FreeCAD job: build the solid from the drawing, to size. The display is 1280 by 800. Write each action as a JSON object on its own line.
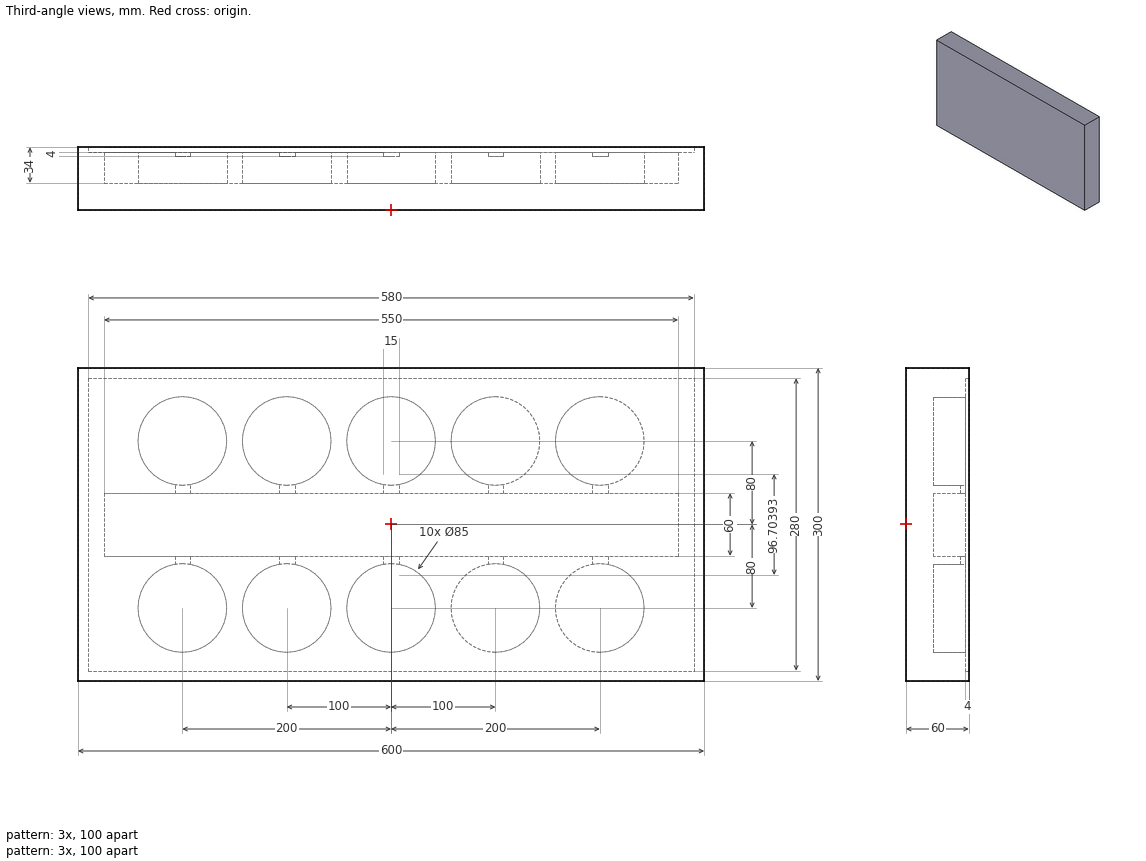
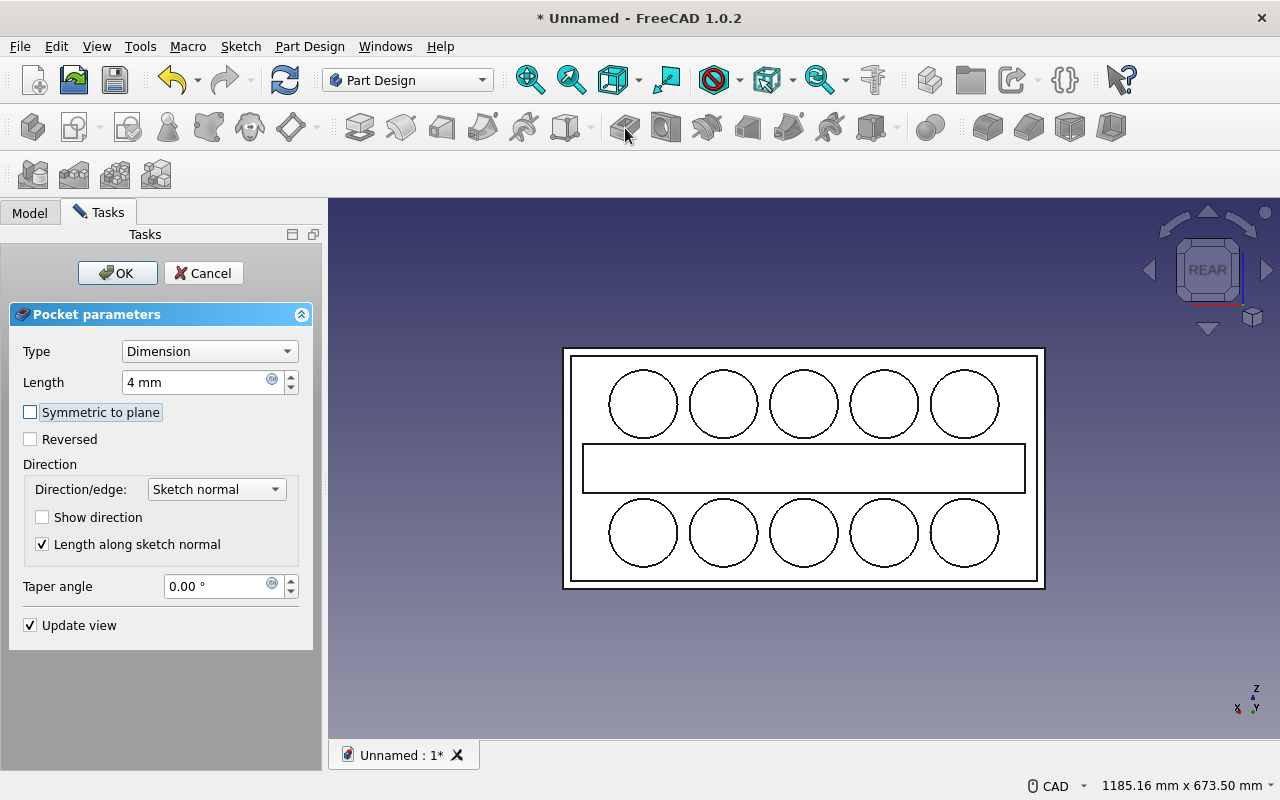
{"action": "left_click", "coordinate": [118, 273]}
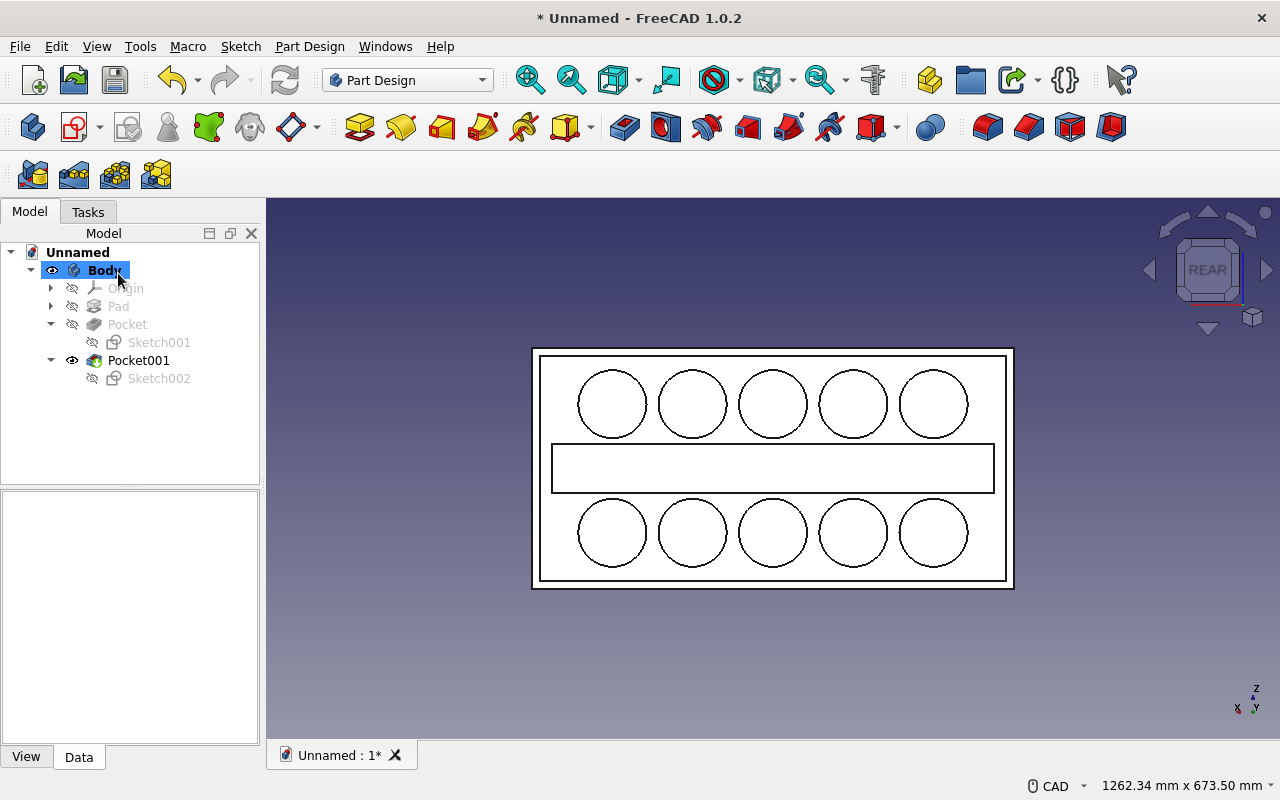
{"action": "left_click", "coordinate": [573, 371]}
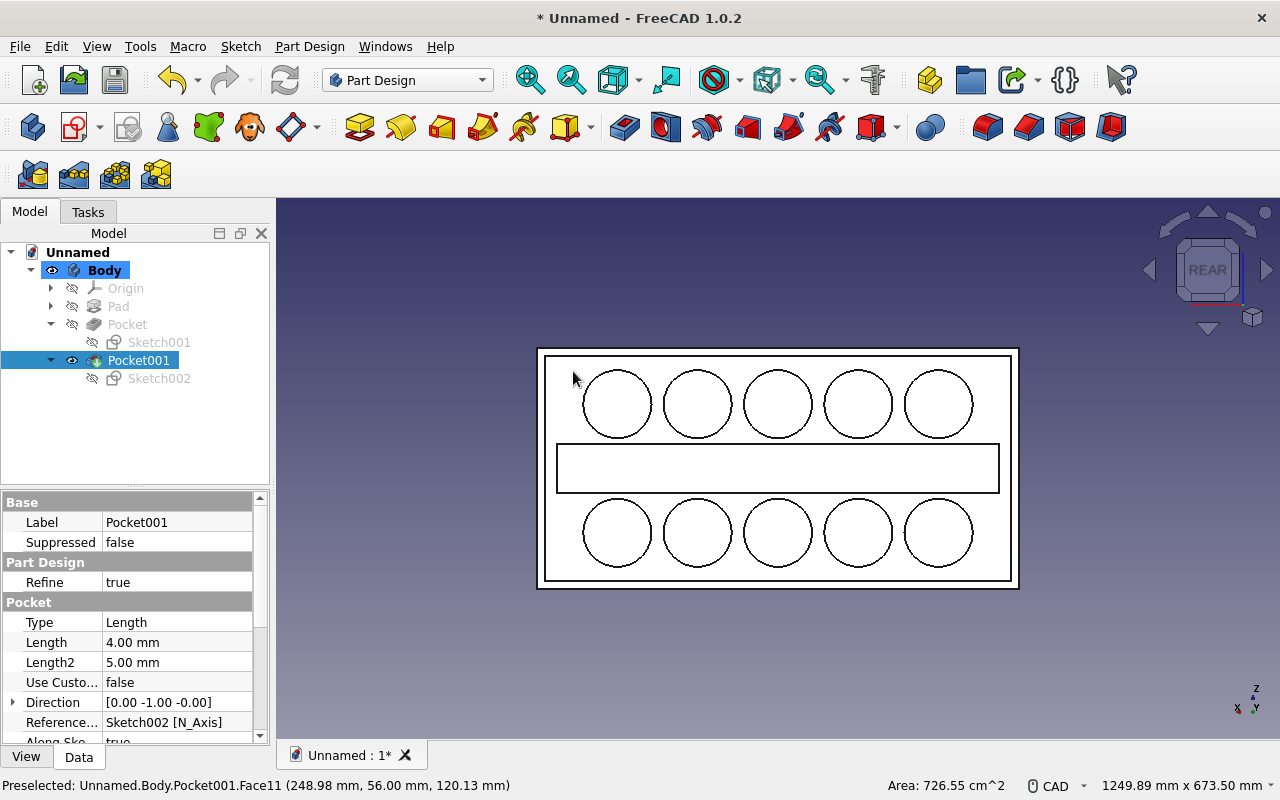
{"action": "left_click", "coordinate": [74, 128]}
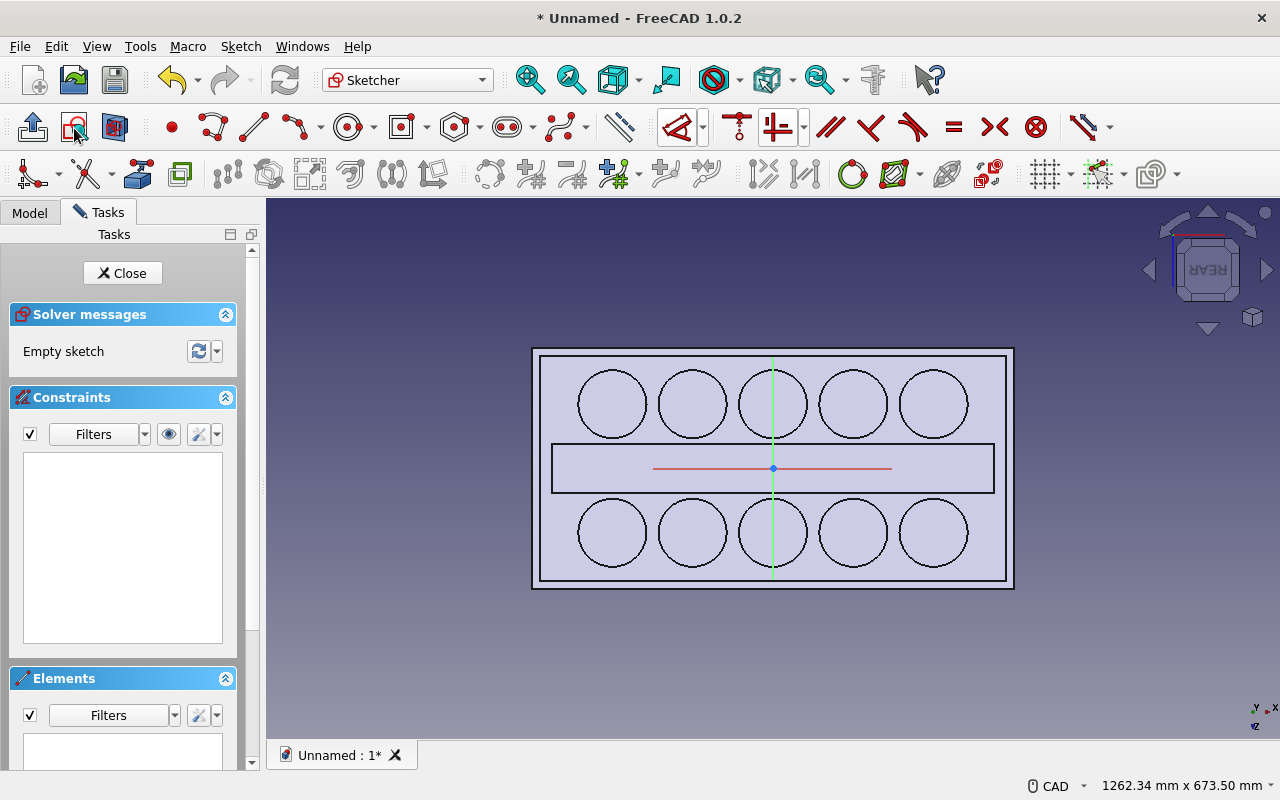
{"action": "left_click", "coordinate": [115, 128]}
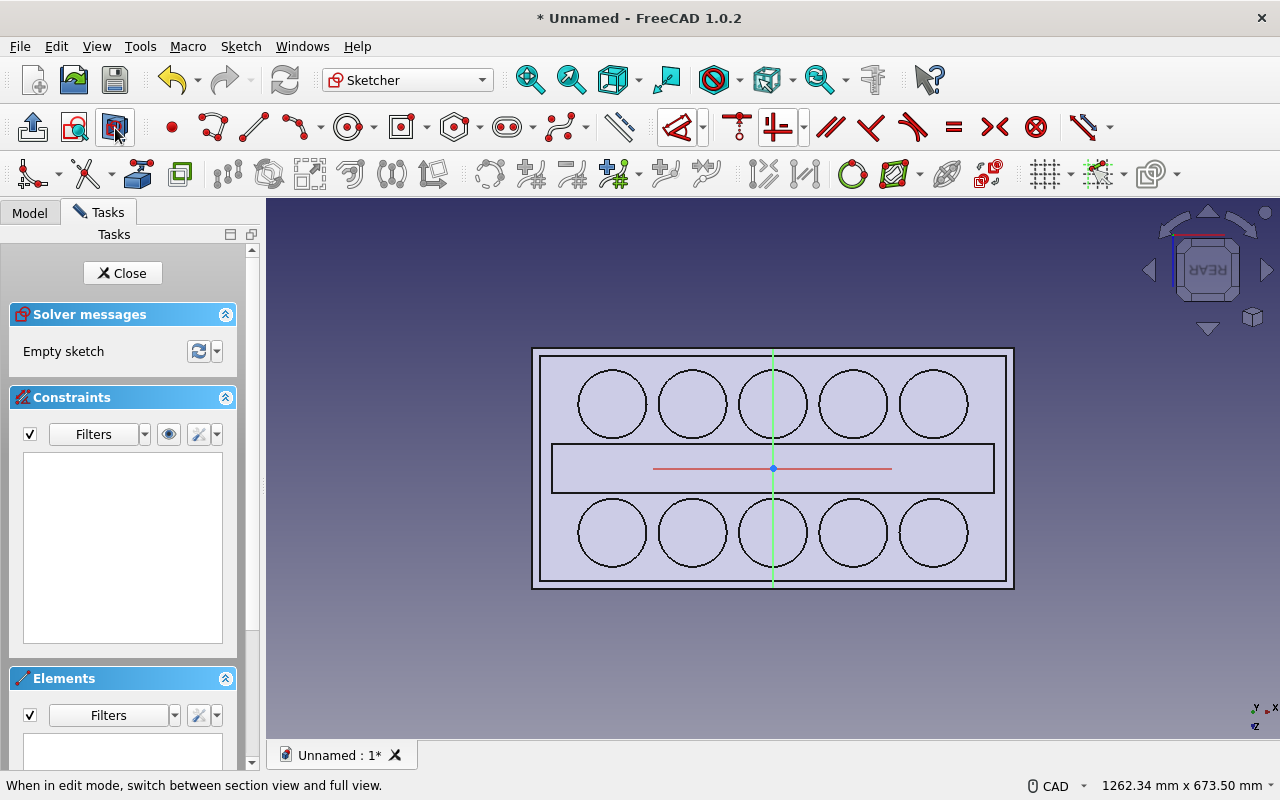
{"action": "scroll", "coordinate": [795, 468], "scroll_direction": "up", "scroll_amount": 7}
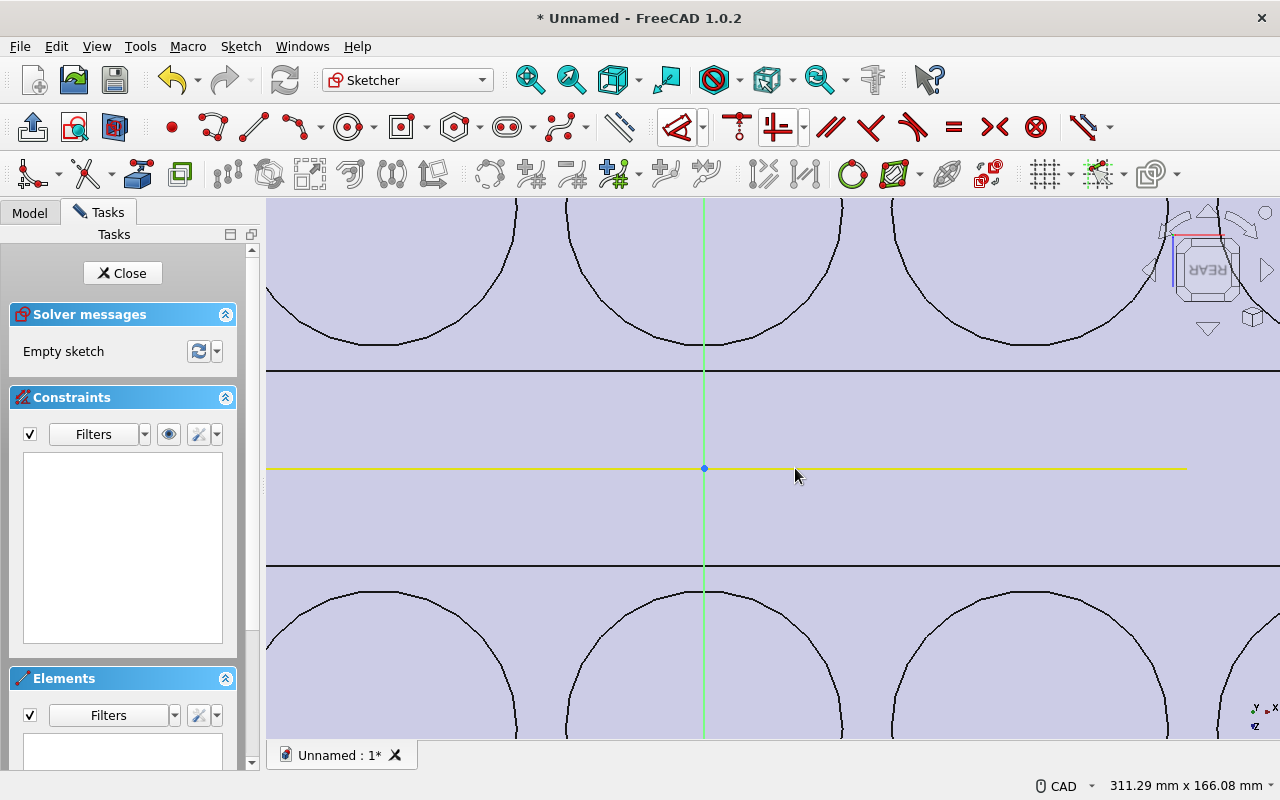
{"action": "left_click", "coordinate": [400, 128]}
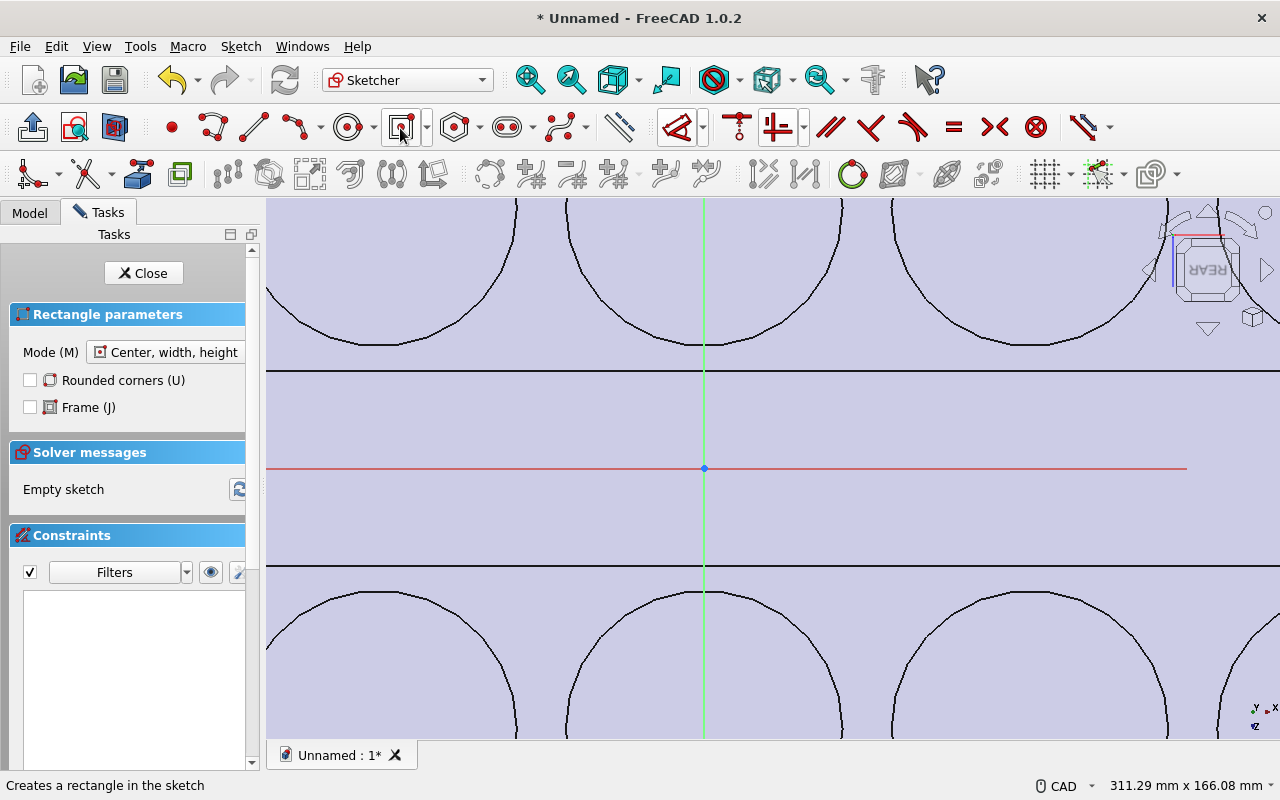
{"action": "left_click", "coordinate": [704, 468]}
{"action": "mouse_move", "coordinate": [729, 311]}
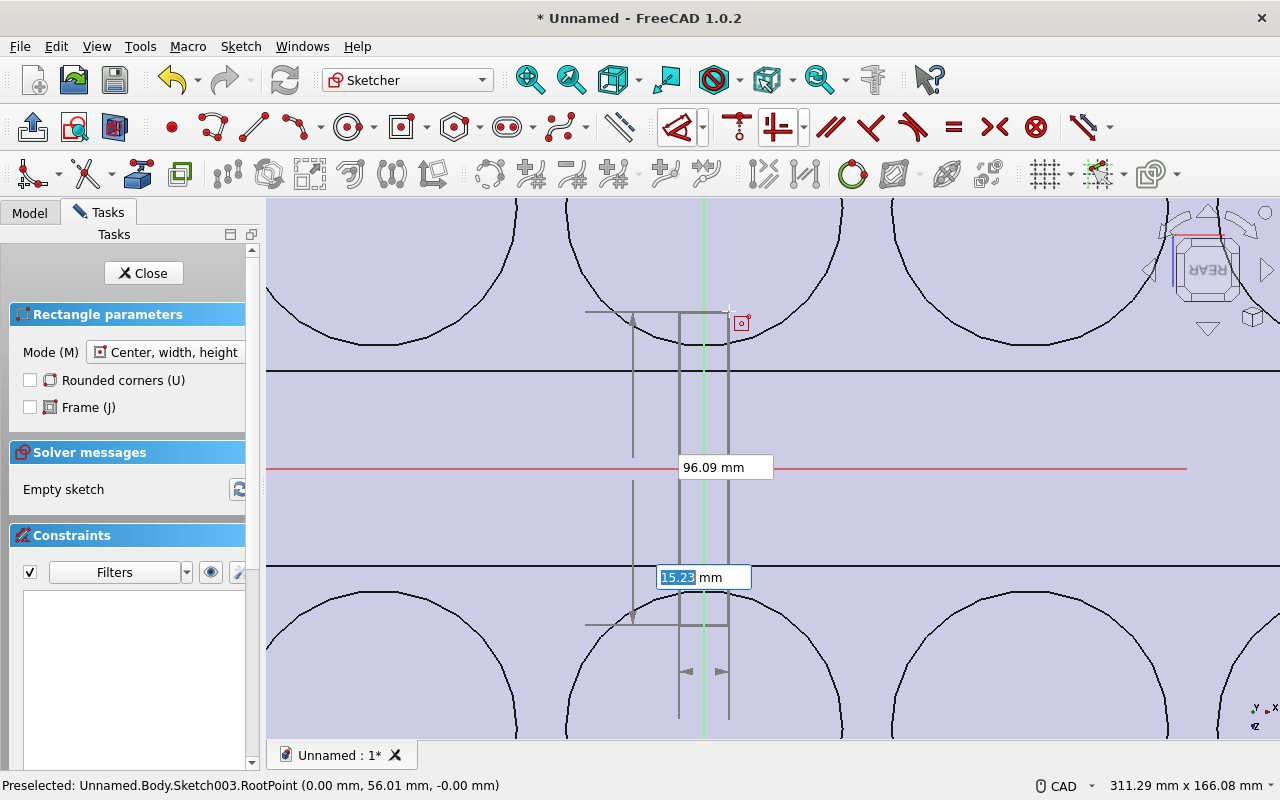
{"action": "type", "text": "15"}
{"action": "key", "text": "Tab"}
{"action": "type", "text": "96.70393"}
{"action": "key", "text": "Return"}
{"action": "key", "text": "Escape"}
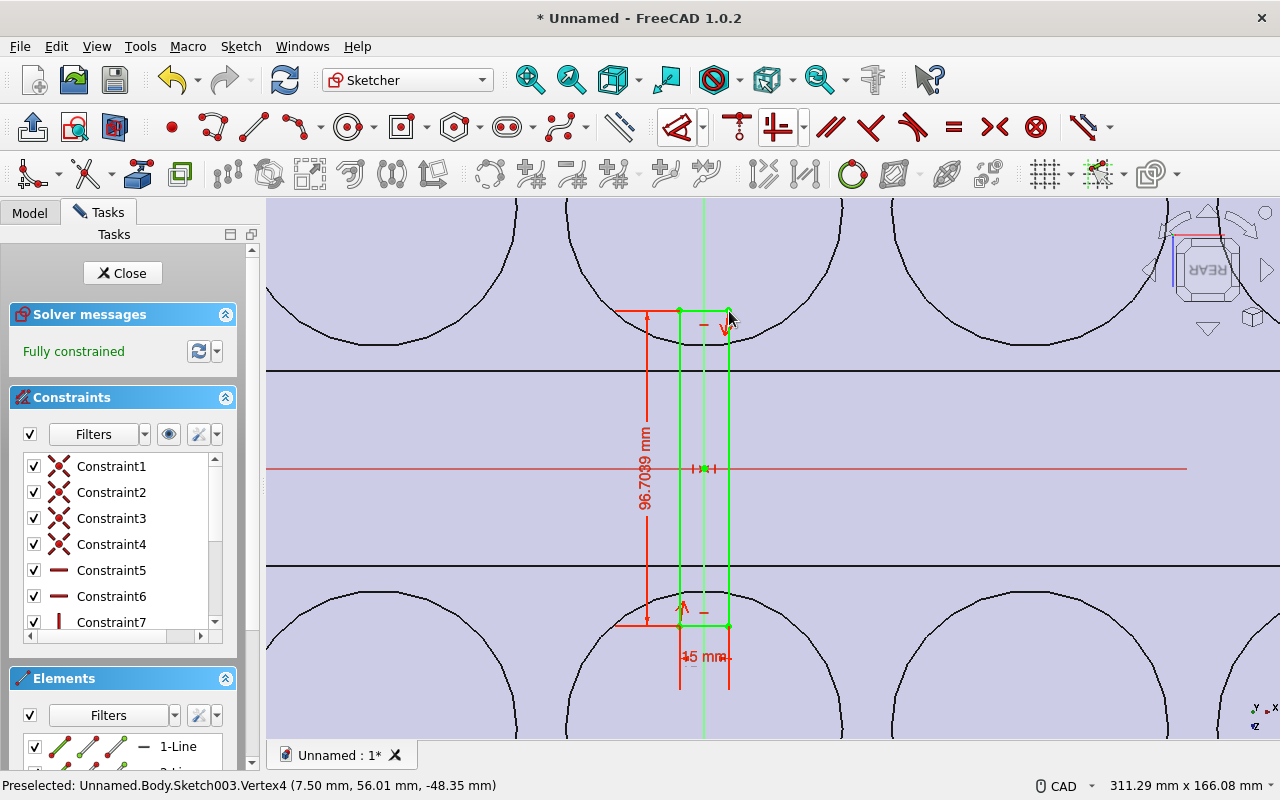
{"action": "left_click", "coordinate": [123, 273]}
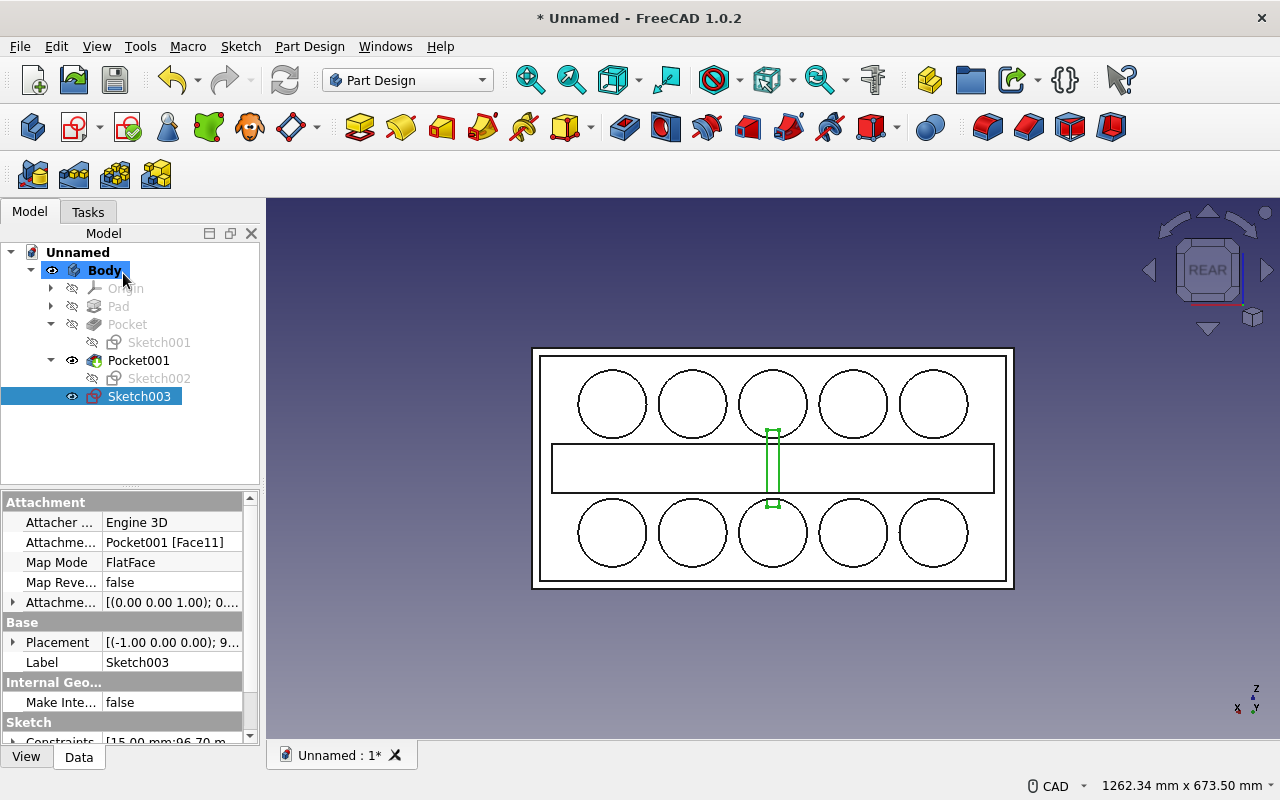
{"action": "left_click", "coordinate": [625, 128]}